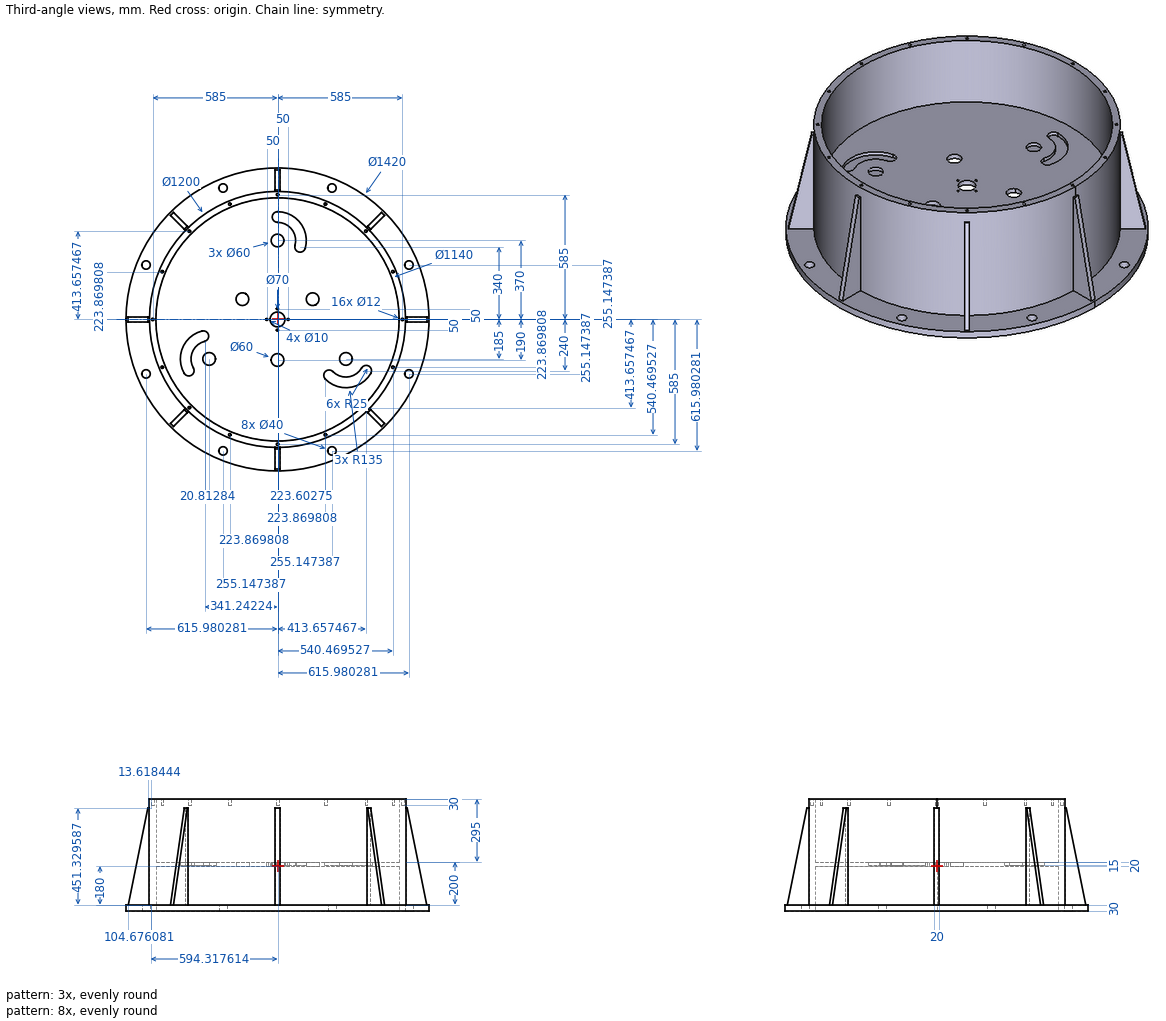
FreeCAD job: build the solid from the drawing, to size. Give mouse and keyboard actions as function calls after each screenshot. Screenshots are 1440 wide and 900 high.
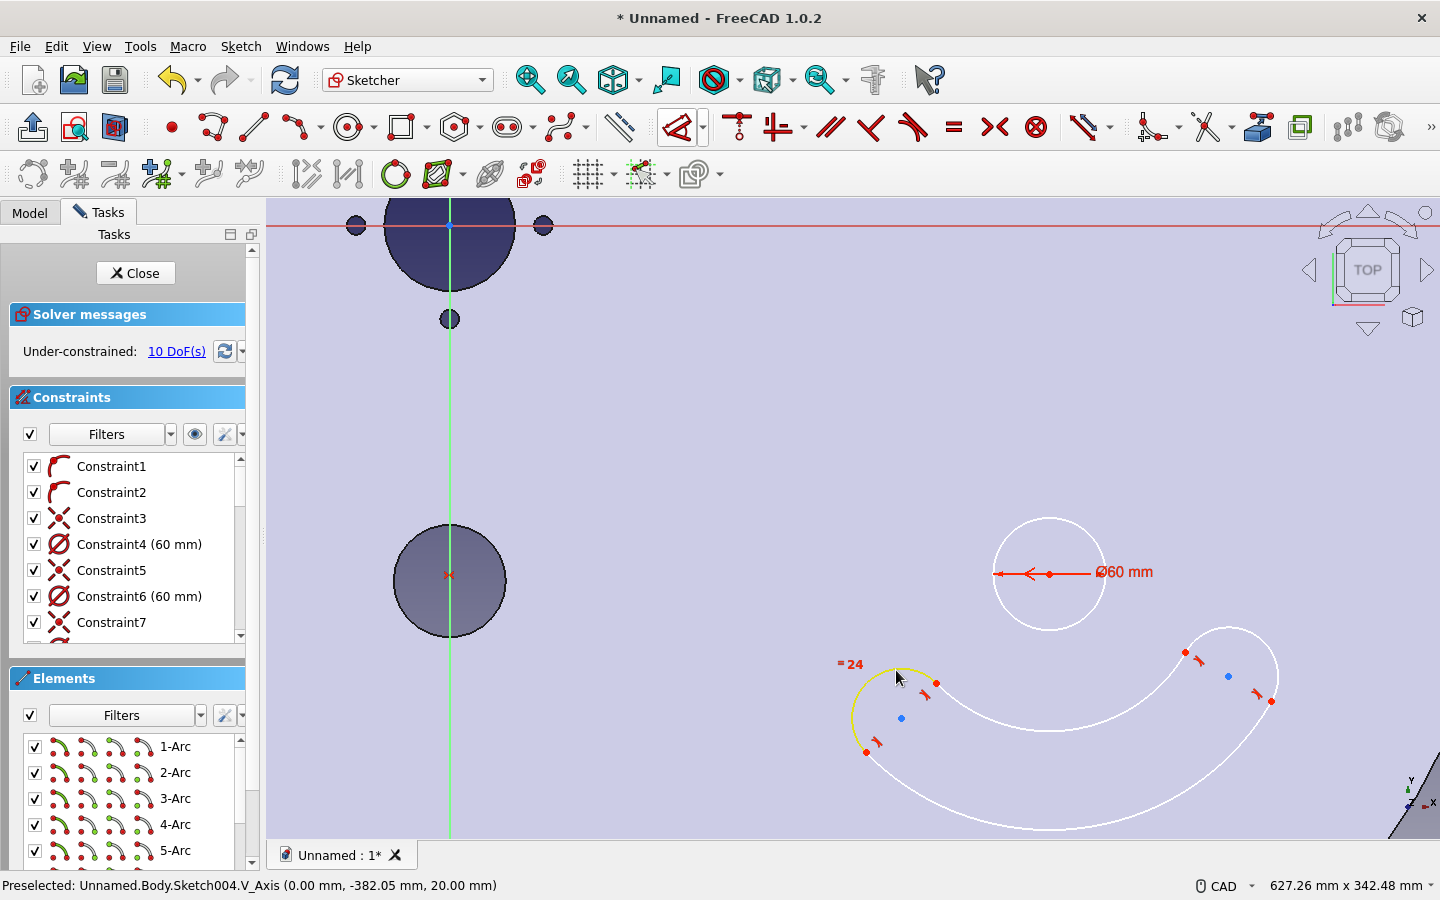
click(894, 669)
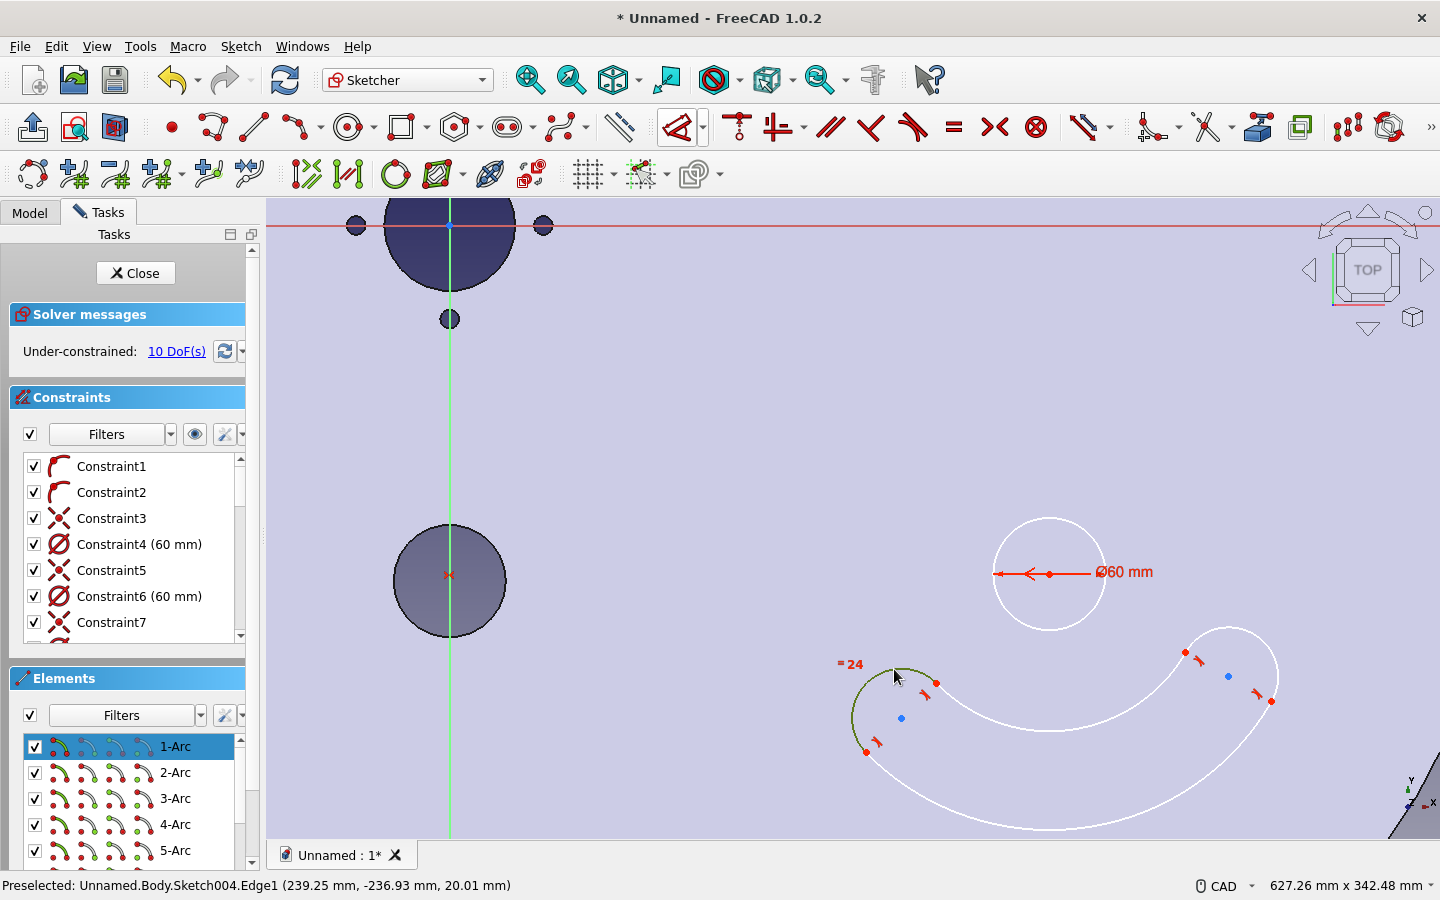
key(k)
key(r)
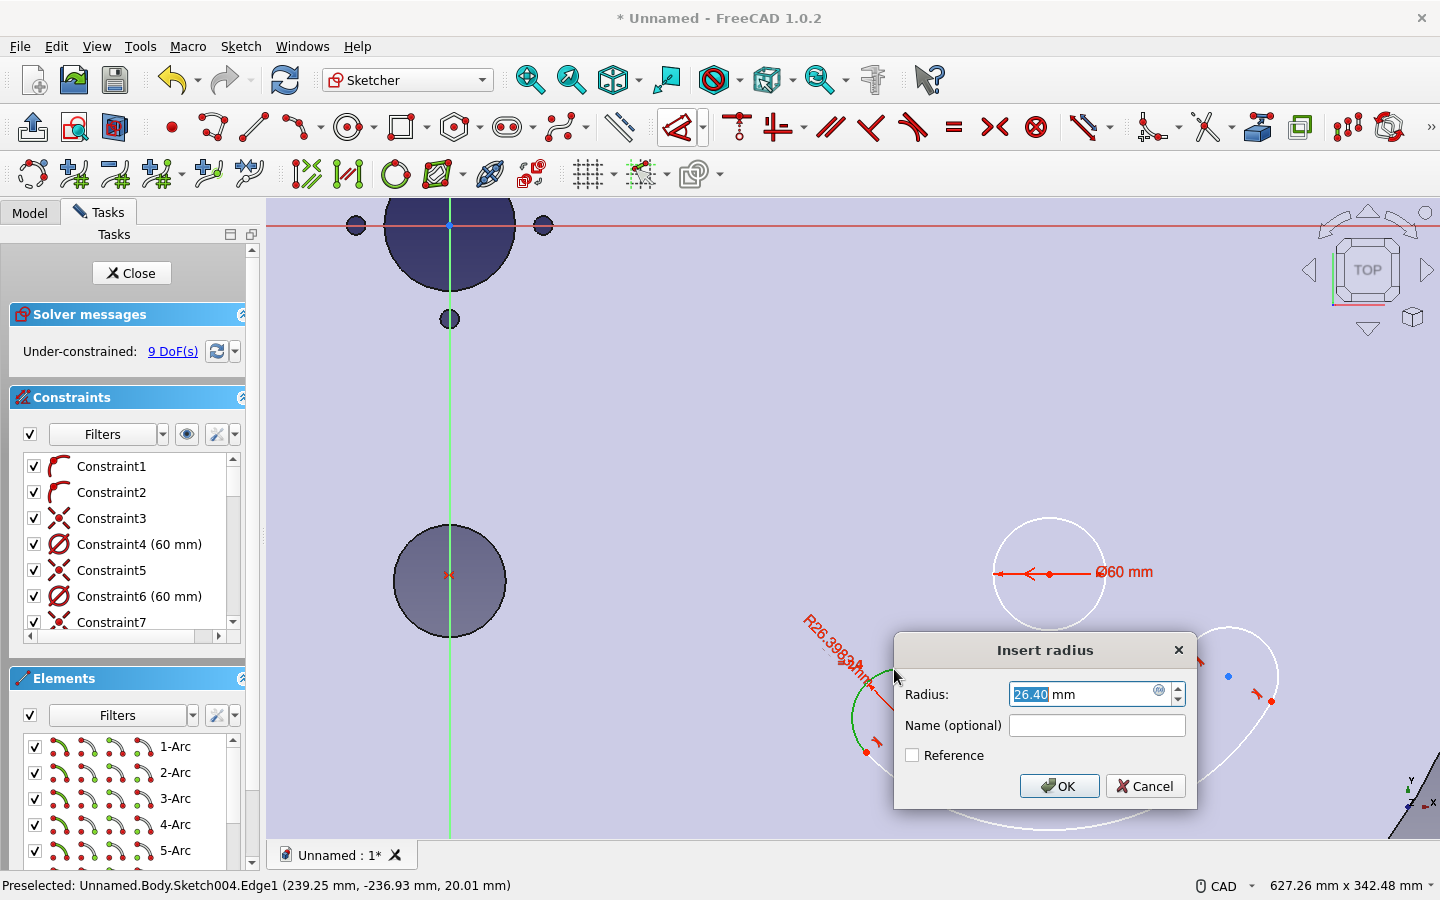
text(25)
key(Return)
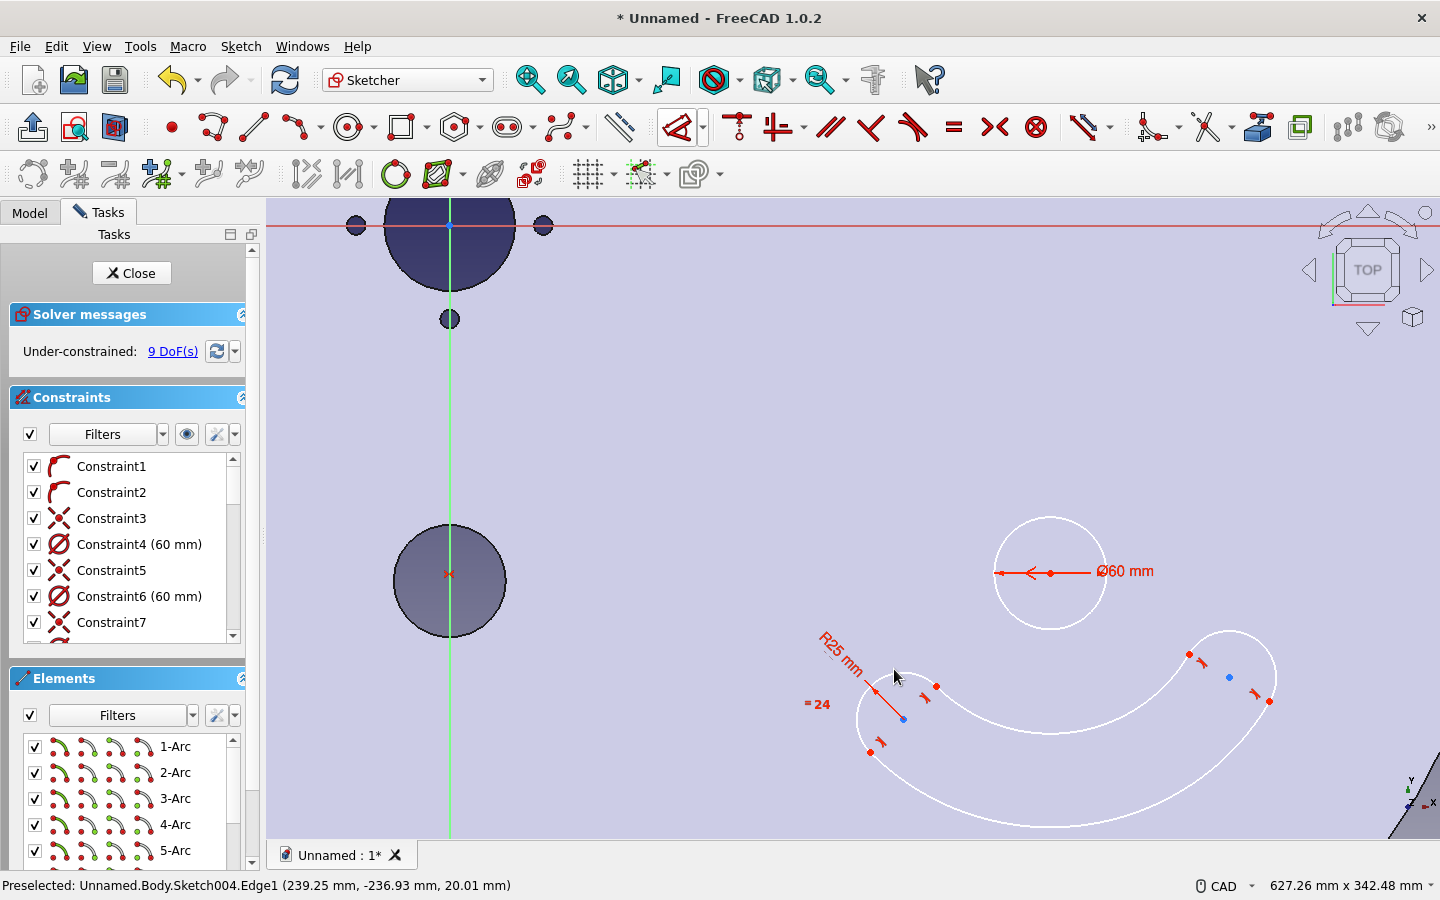
scroll(896, 671, down, 7)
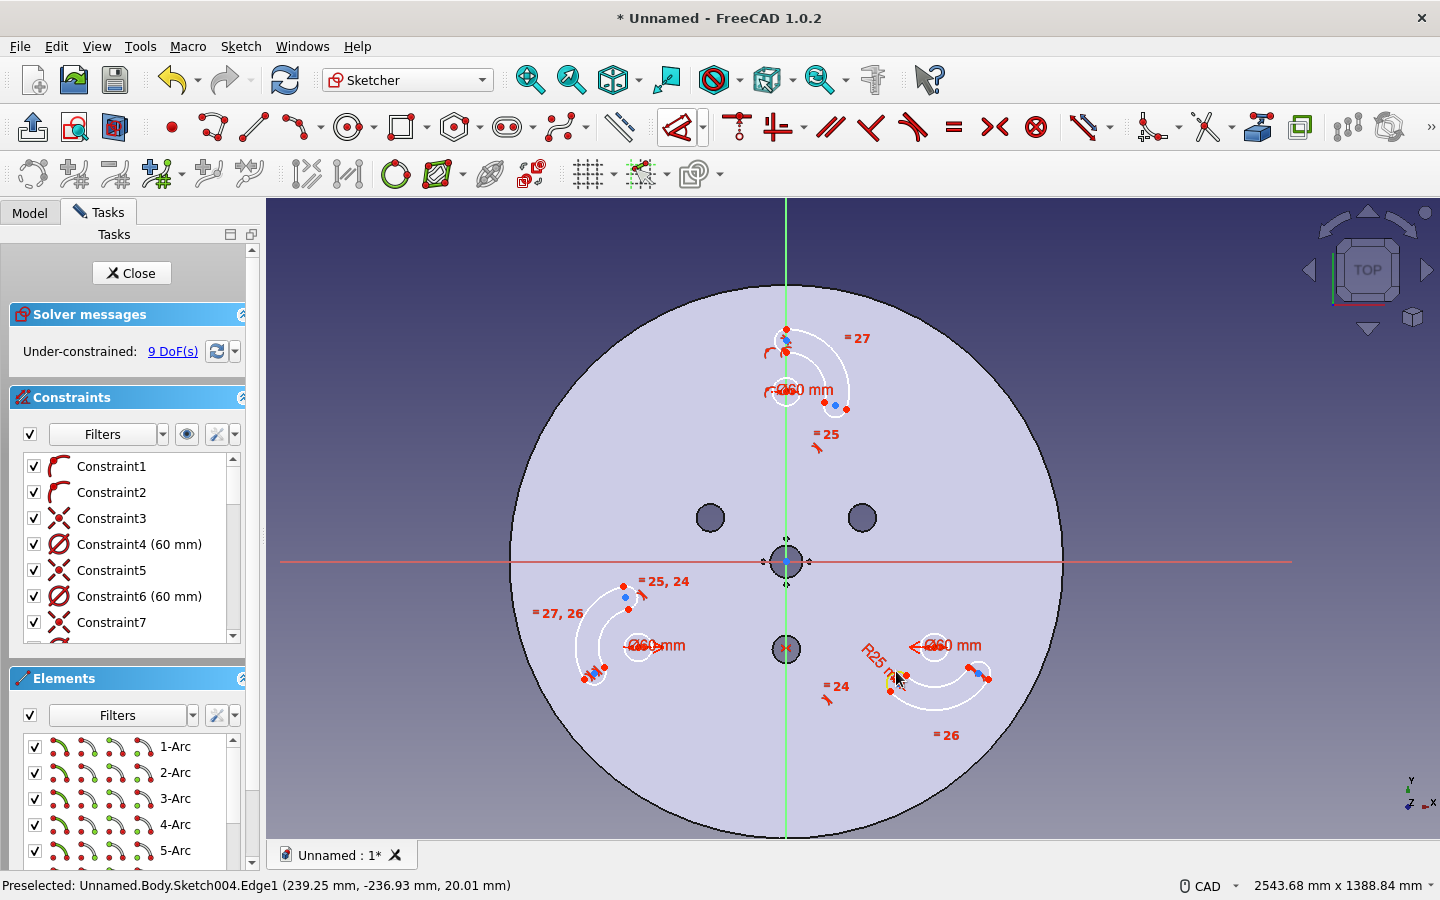
click(964, 703)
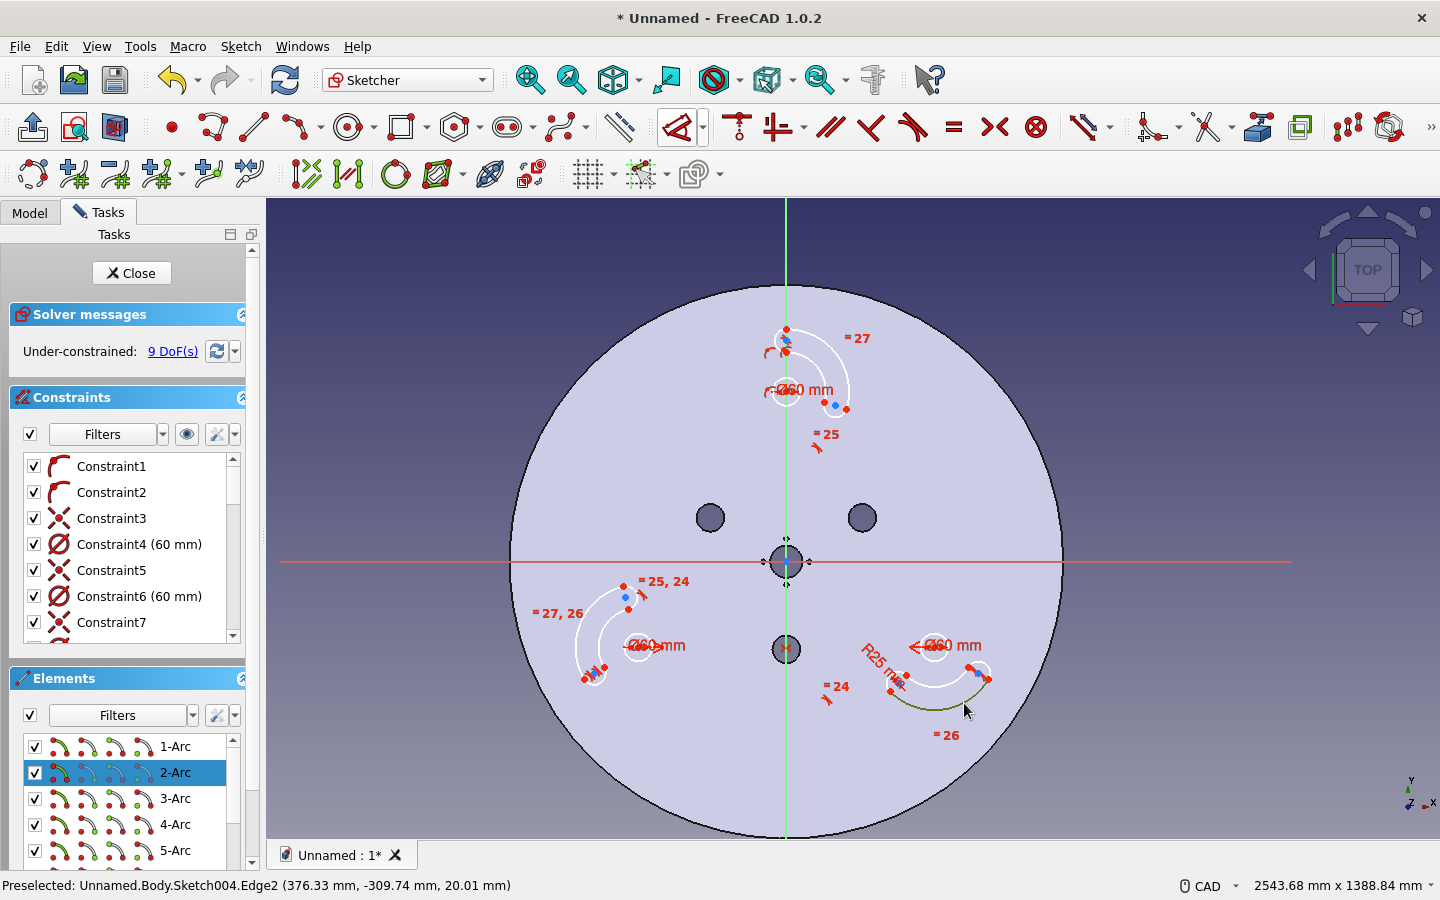
key(k)
key(r)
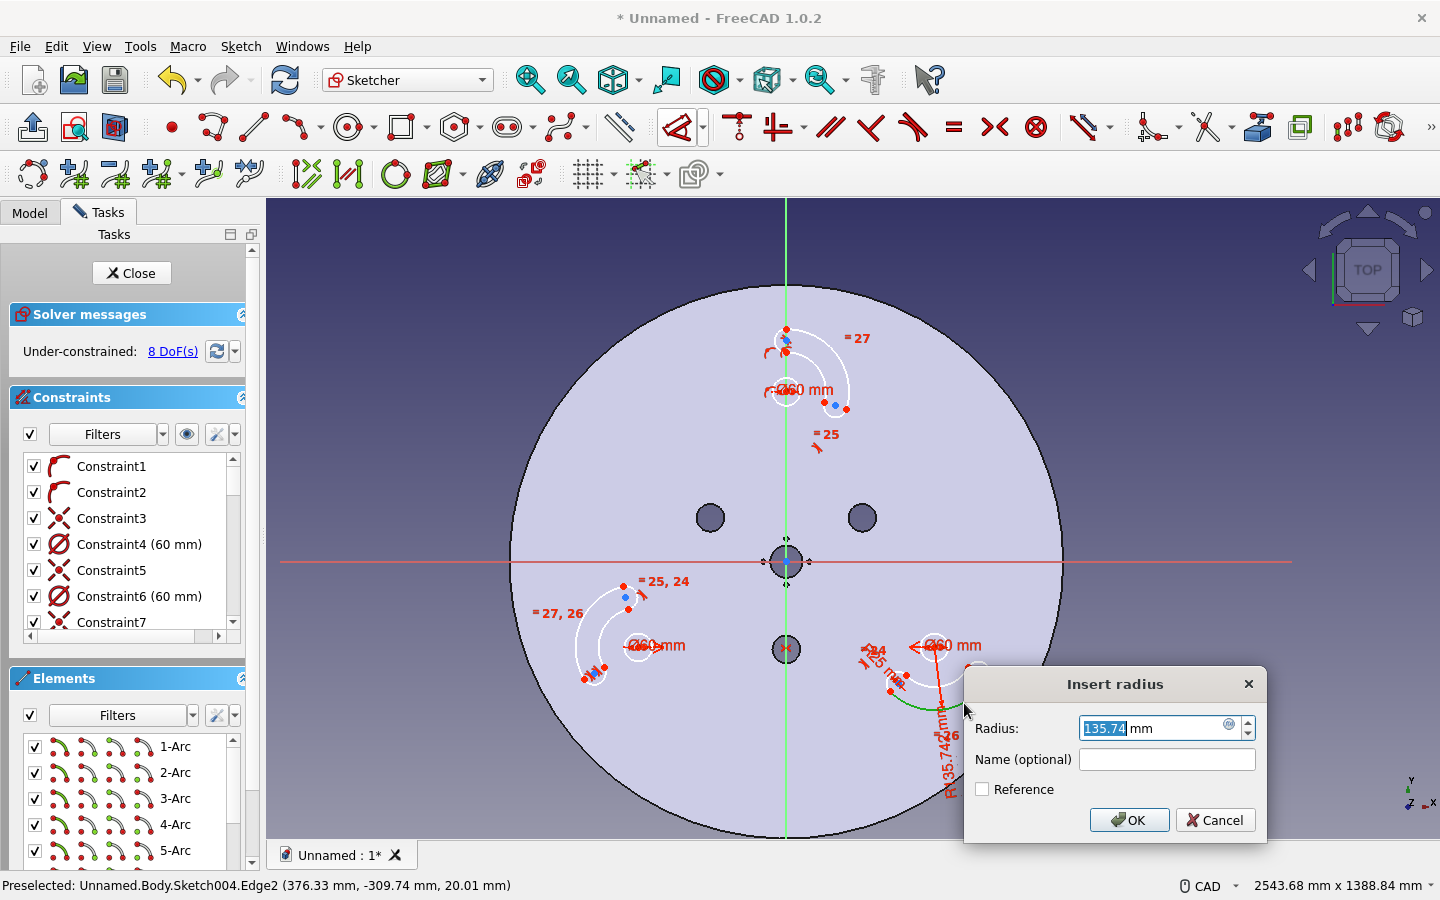
text(135)
key(Return)